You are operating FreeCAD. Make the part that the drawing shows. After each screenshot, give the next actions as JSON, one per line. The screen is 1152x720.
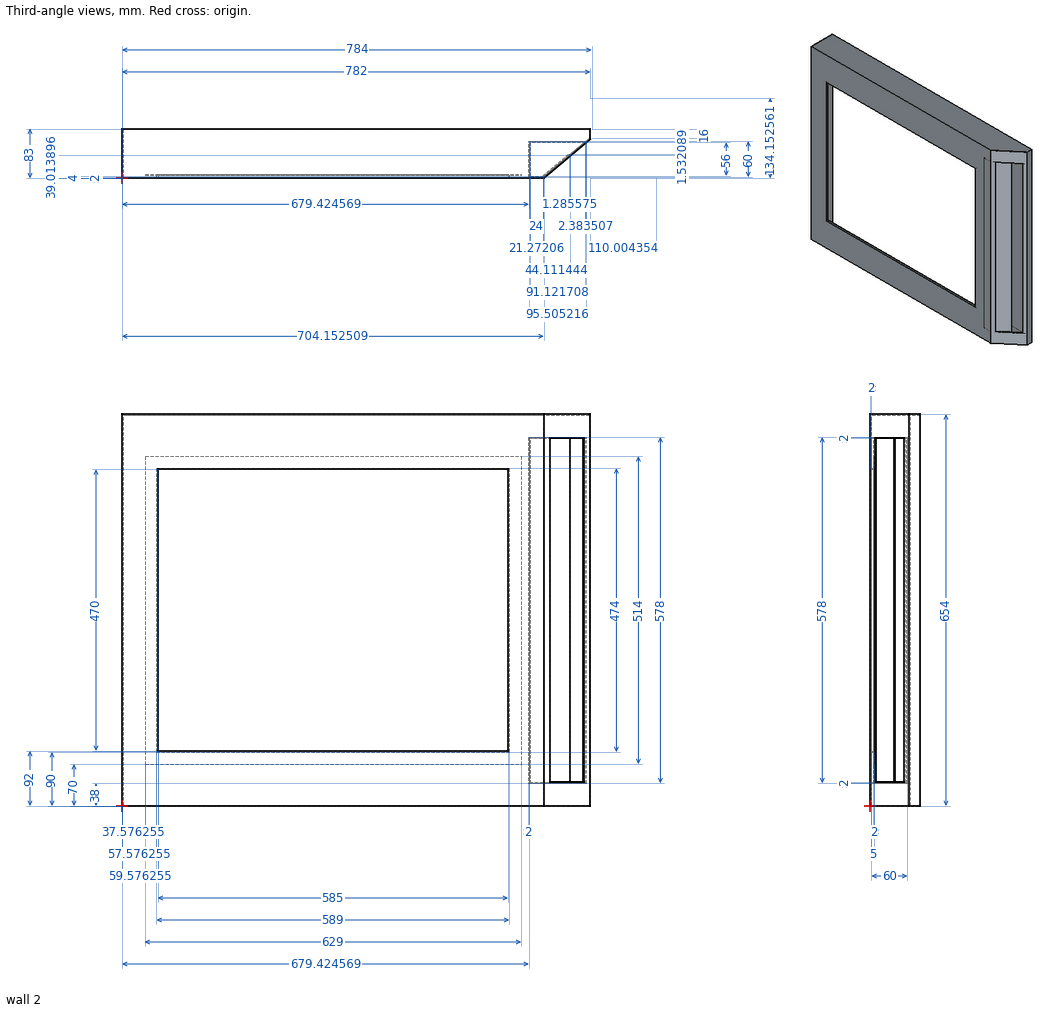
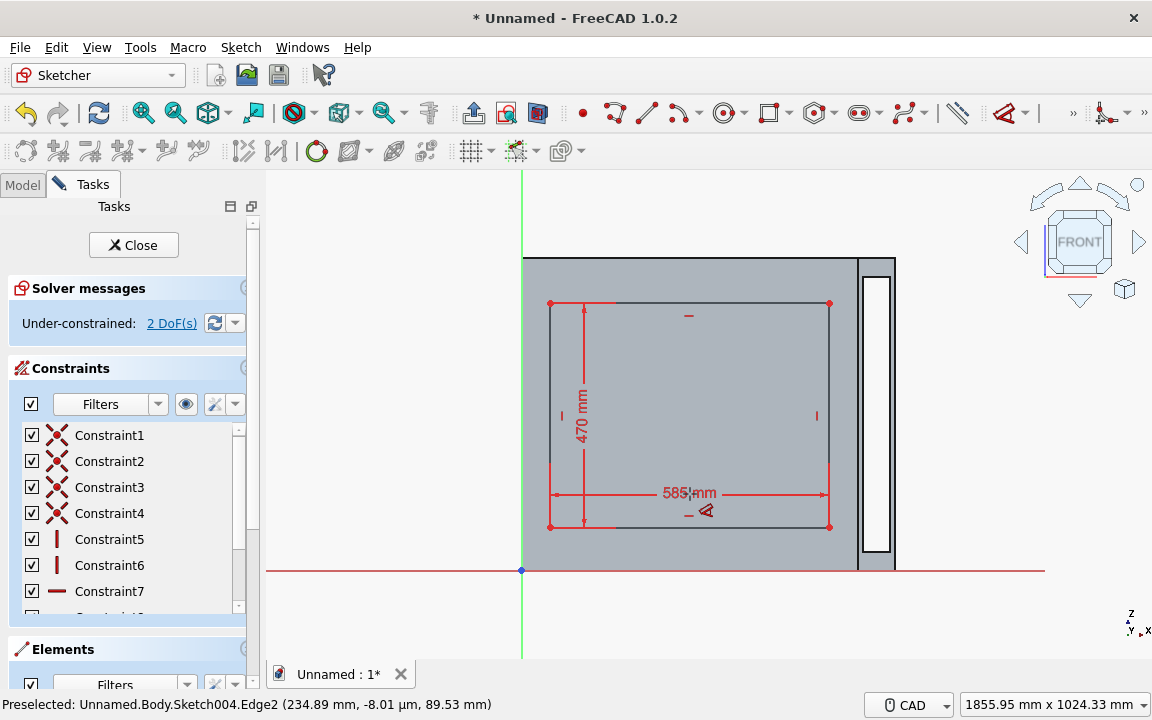
{"action": "left_click", "coordinate": [550, 528]}
{"action": "left_click", "coordinate": [488, 549]}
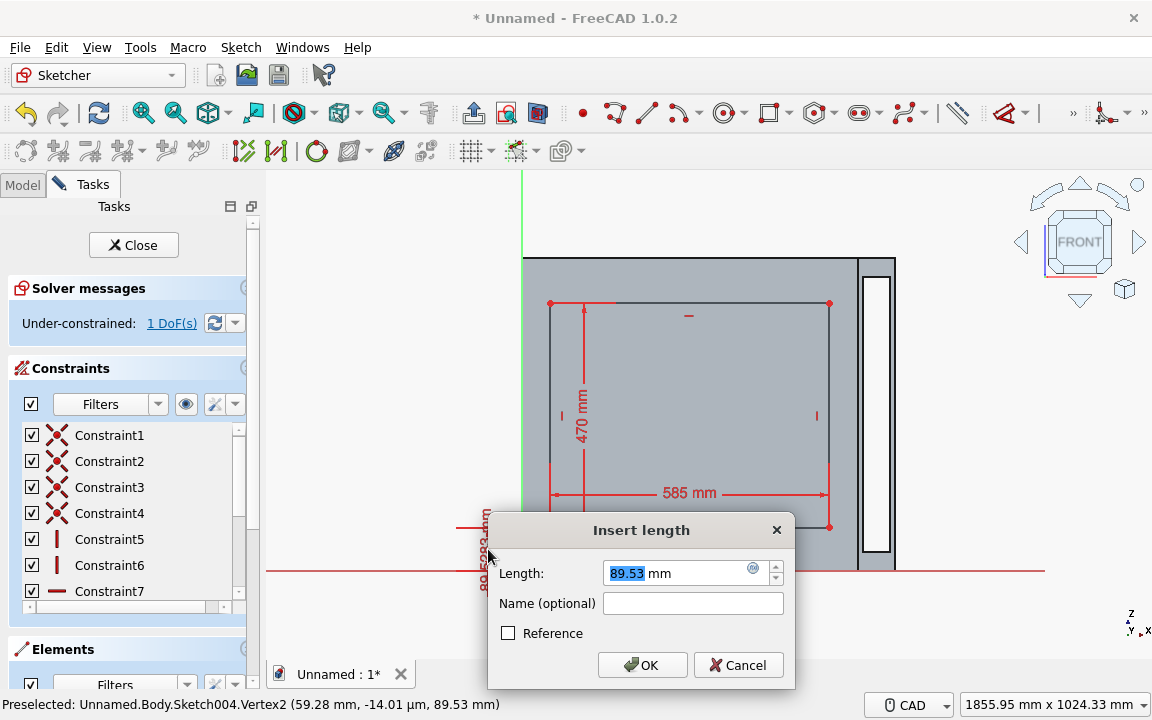
{"action": "type", "text": "92"}
{"action": "key", "text": "Return"}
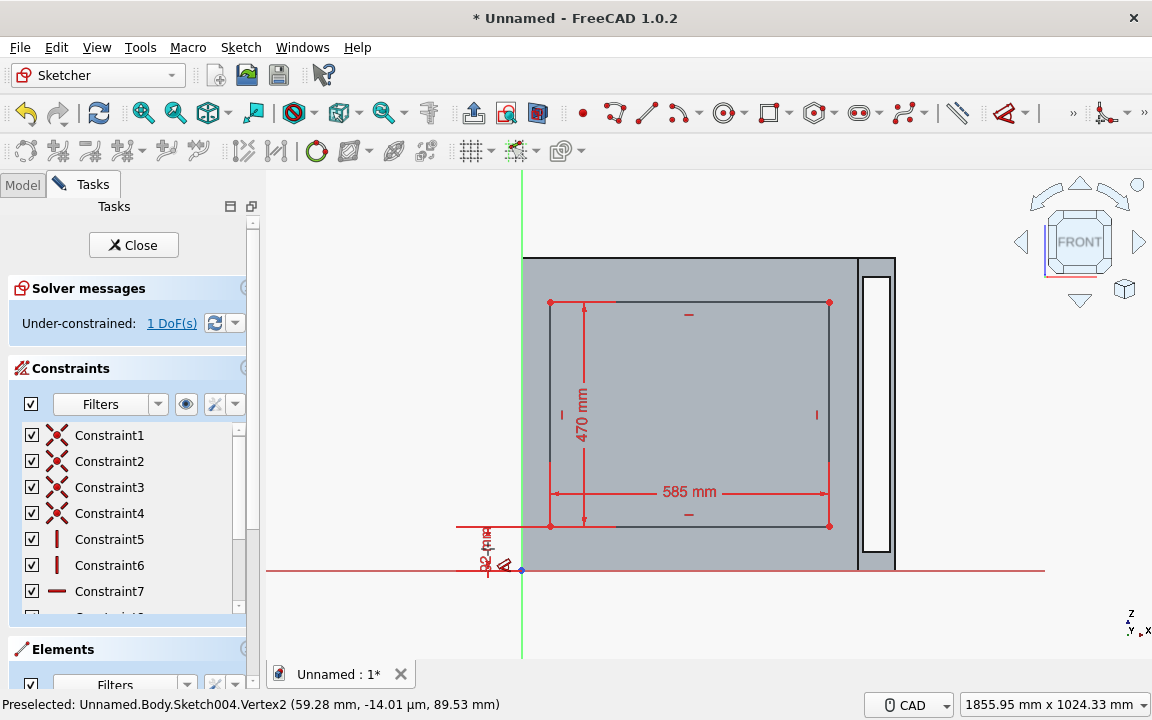
{"action": "scroll", "coordinate": [550, 302], "scroll_direction": "up", "scroll_amount": 2}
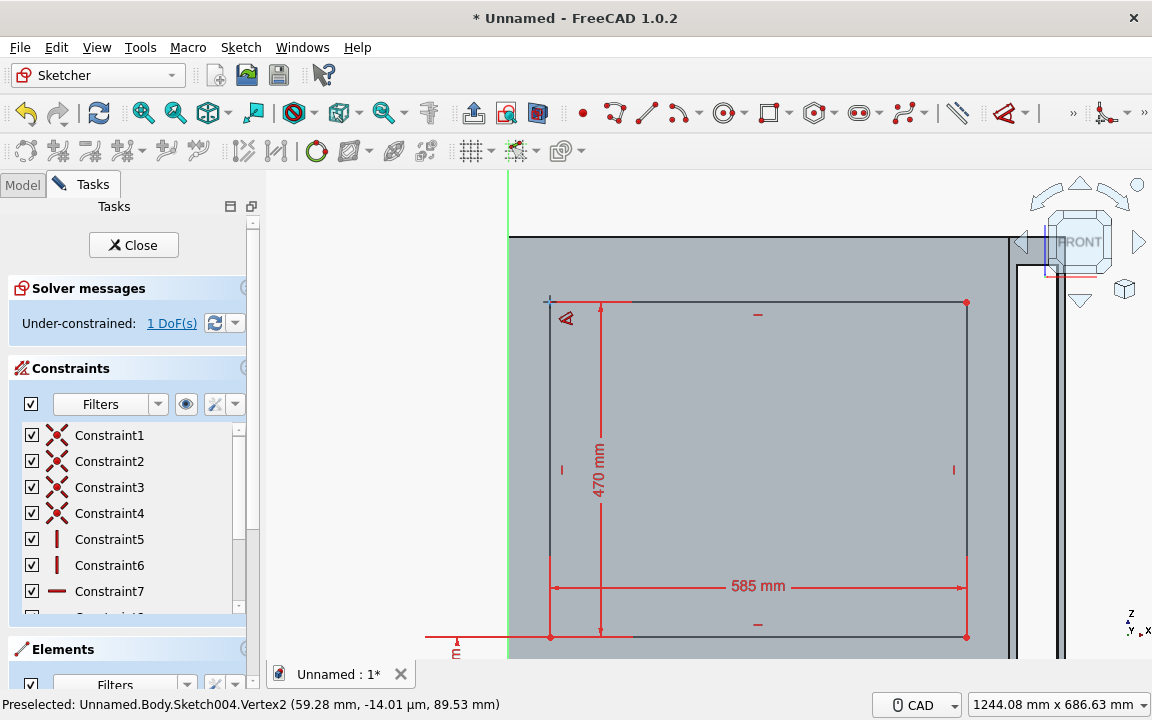
{"action": "left_click", "coordinate": [550, 302]}
{"action": "left_click", "coordinate": [529, 268]}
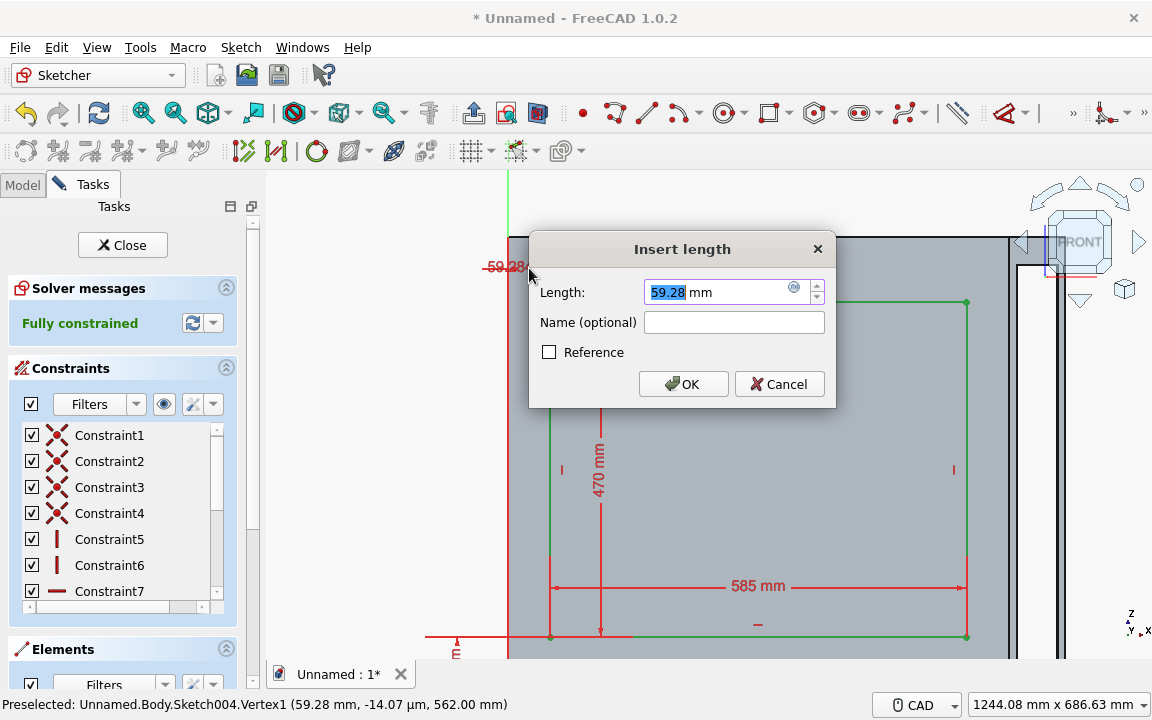
{"action": "type", "text": "59.576255"}
{"action": "key", "text": "Return"}
{"action": "key", "text": "Escape"}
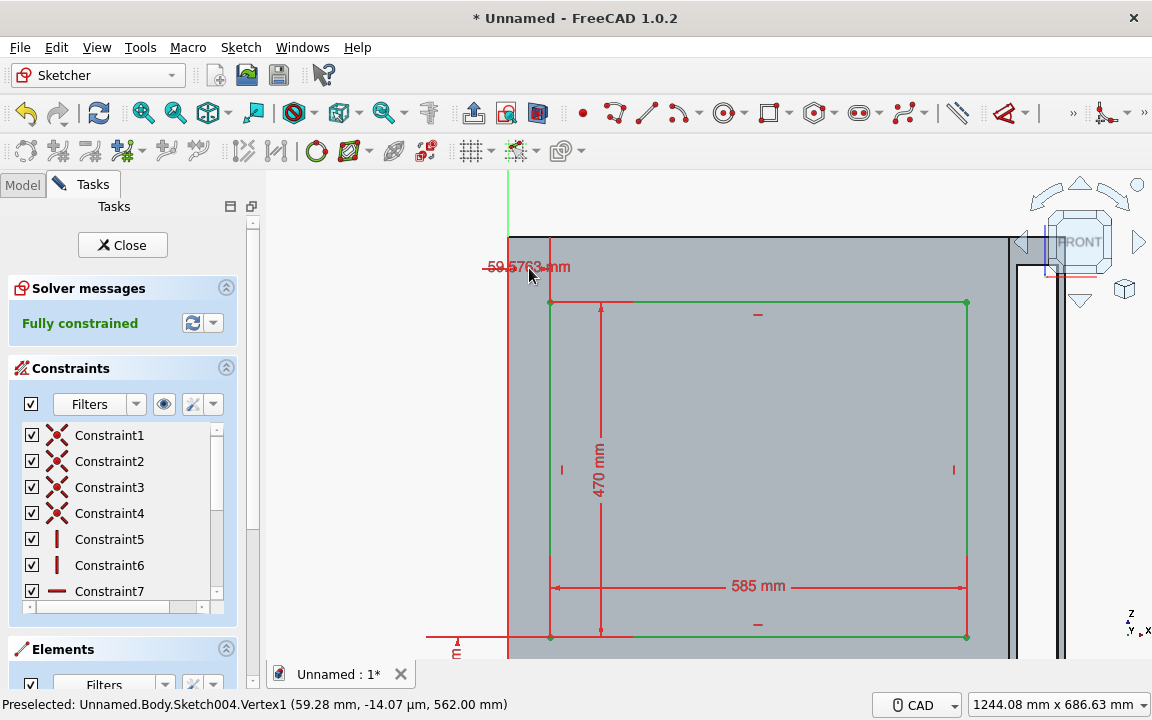
{"action": "left_click", "coordinate": [123, 245]}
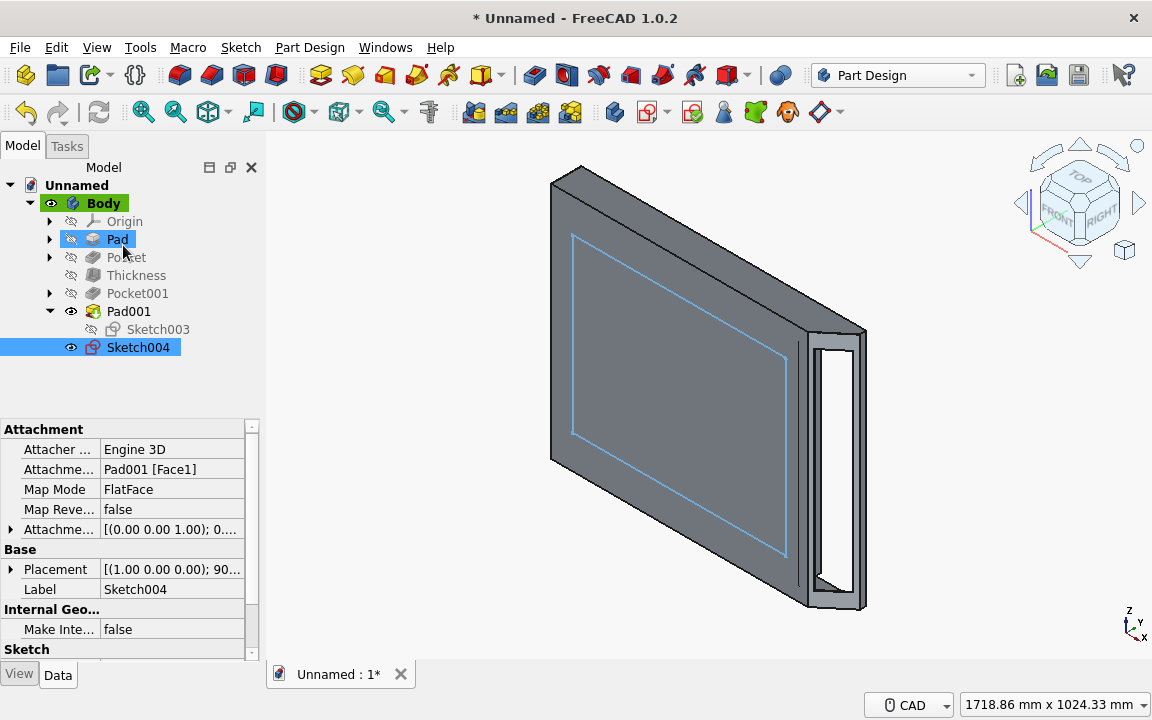
{"action": "left_click", "coordinate": [536, 76]}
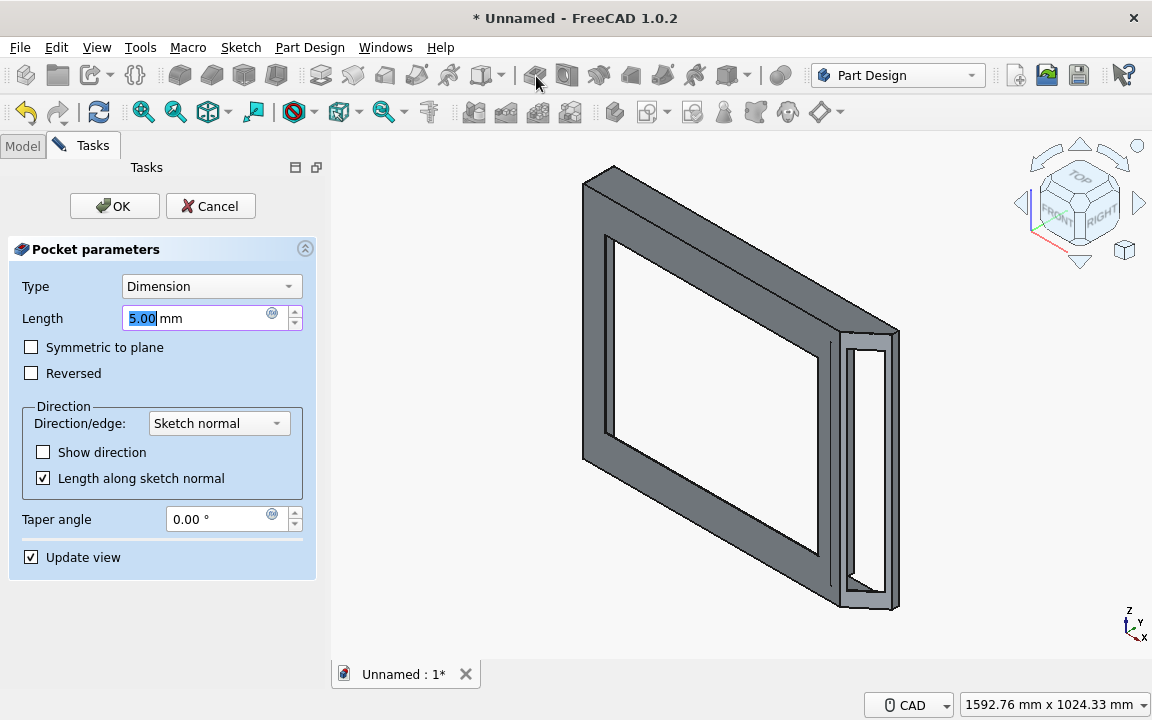
{"action": "type", "text": "2"}
{"action": "key", "text": "Tab"}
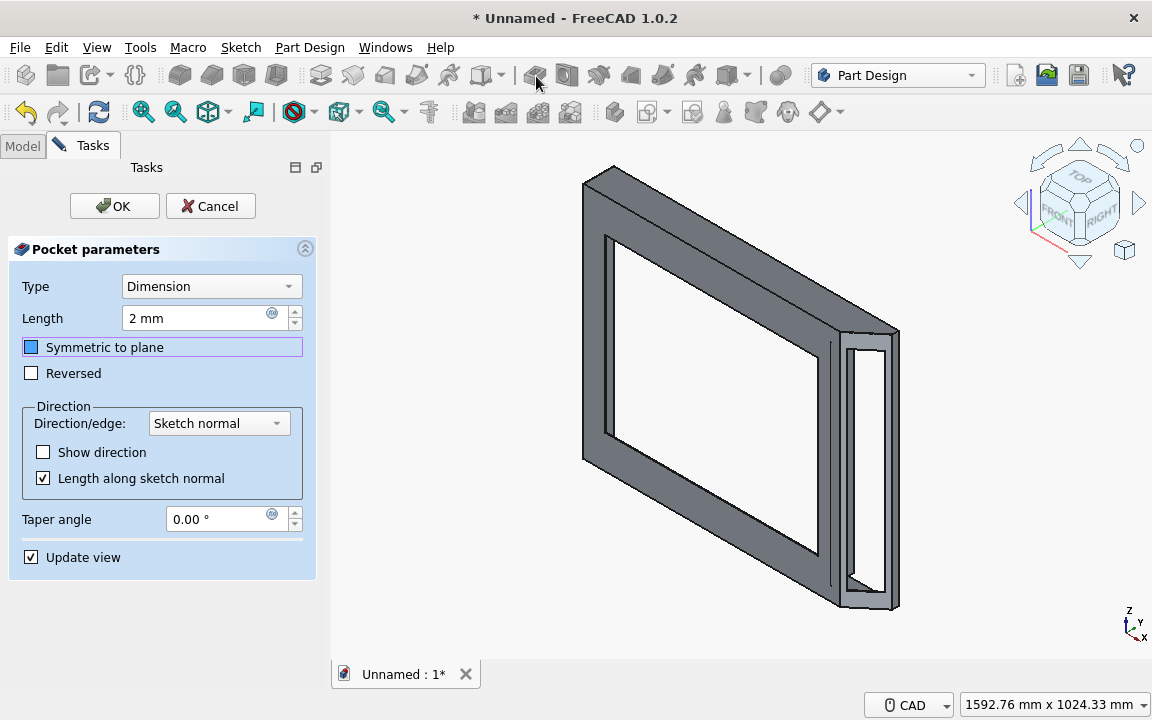
{"action": "left_click", "coordinate": [115, 206]}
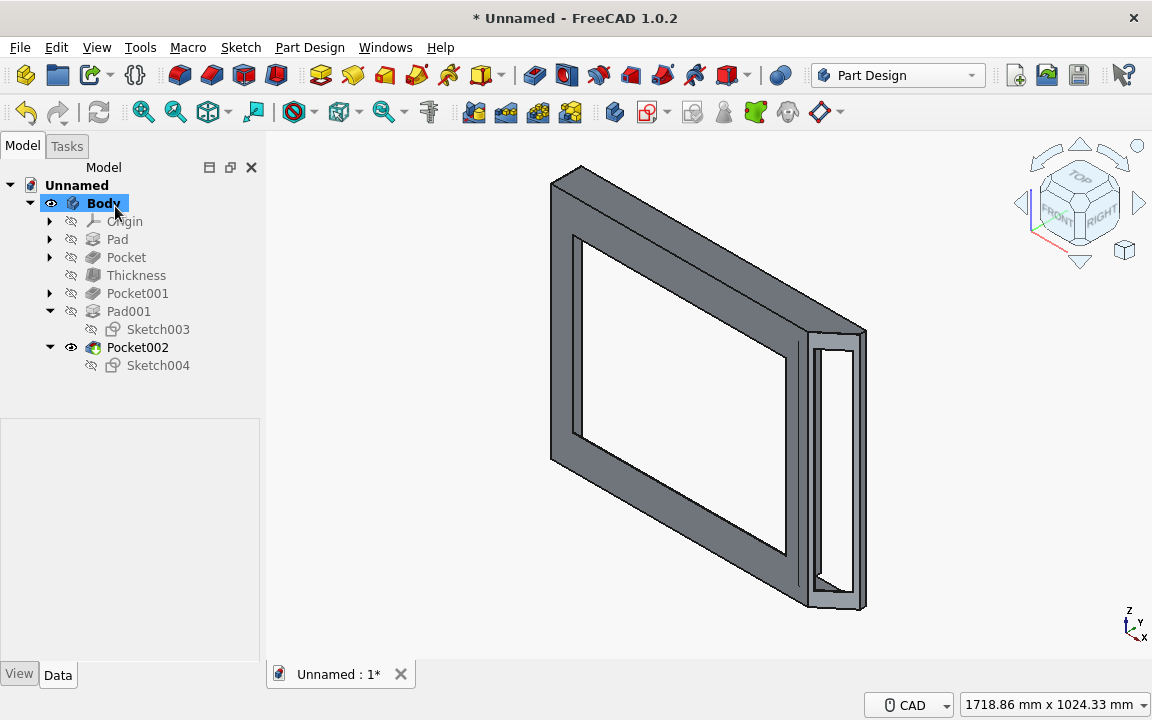
{"action": "key", "text": "4"}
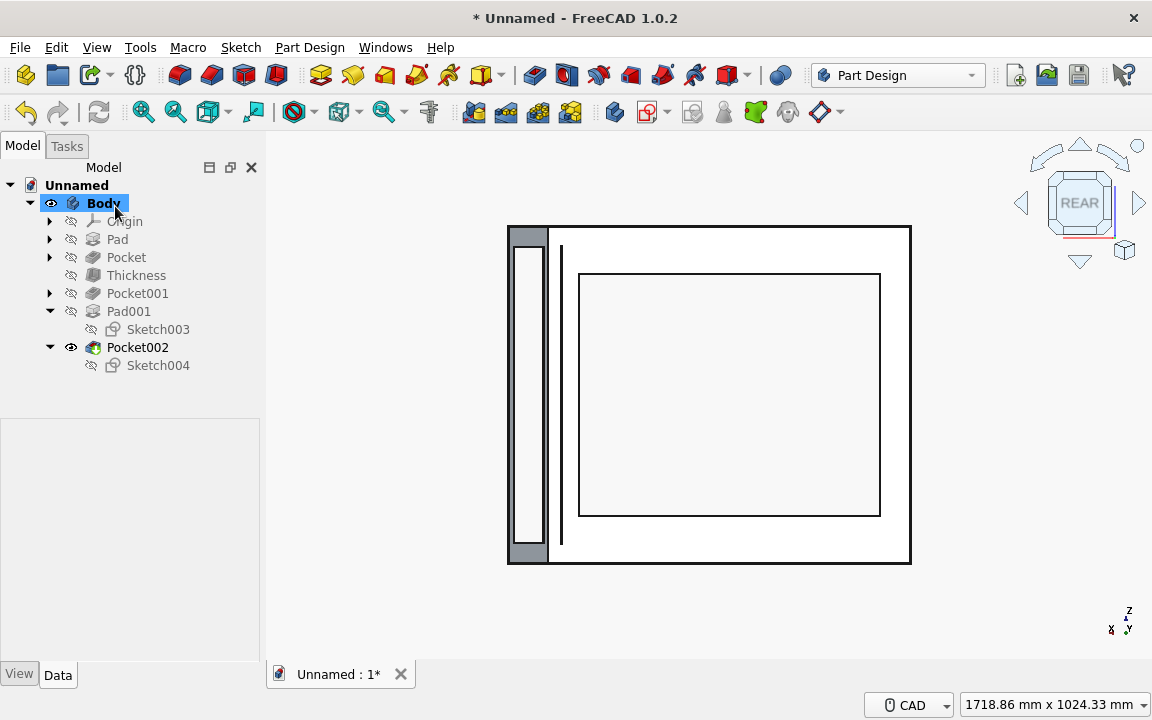
{"action": "left_click", "coordinate": [884, 538]}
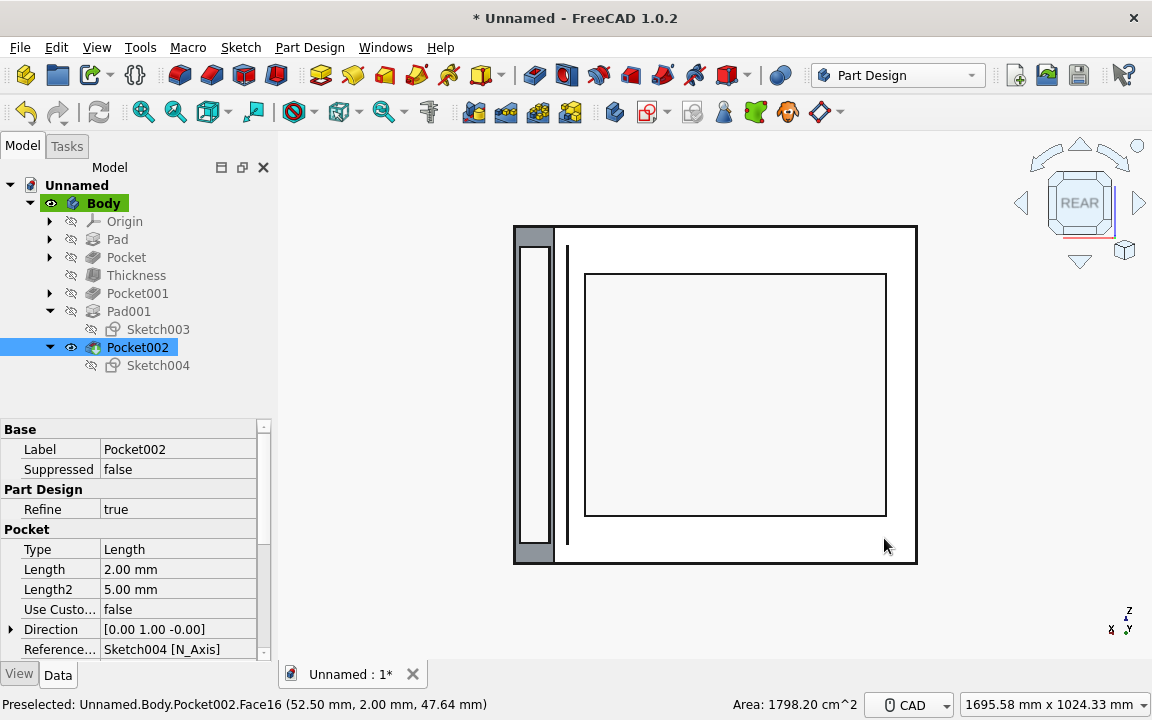
{"action": "left_click", "coordinate": [648, 112]}